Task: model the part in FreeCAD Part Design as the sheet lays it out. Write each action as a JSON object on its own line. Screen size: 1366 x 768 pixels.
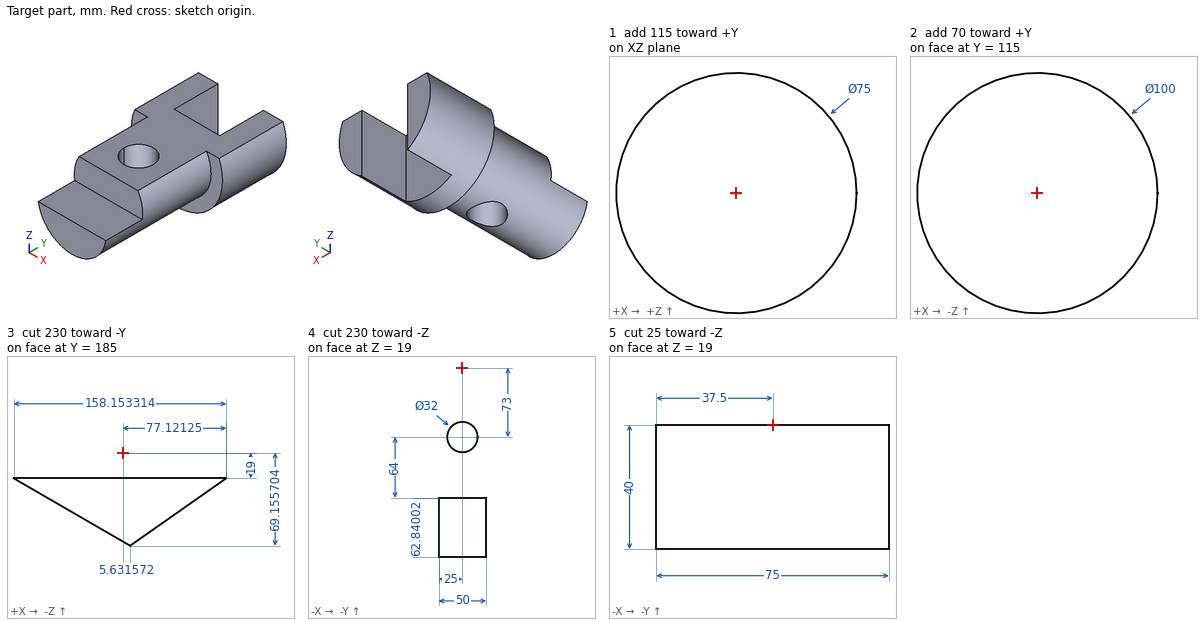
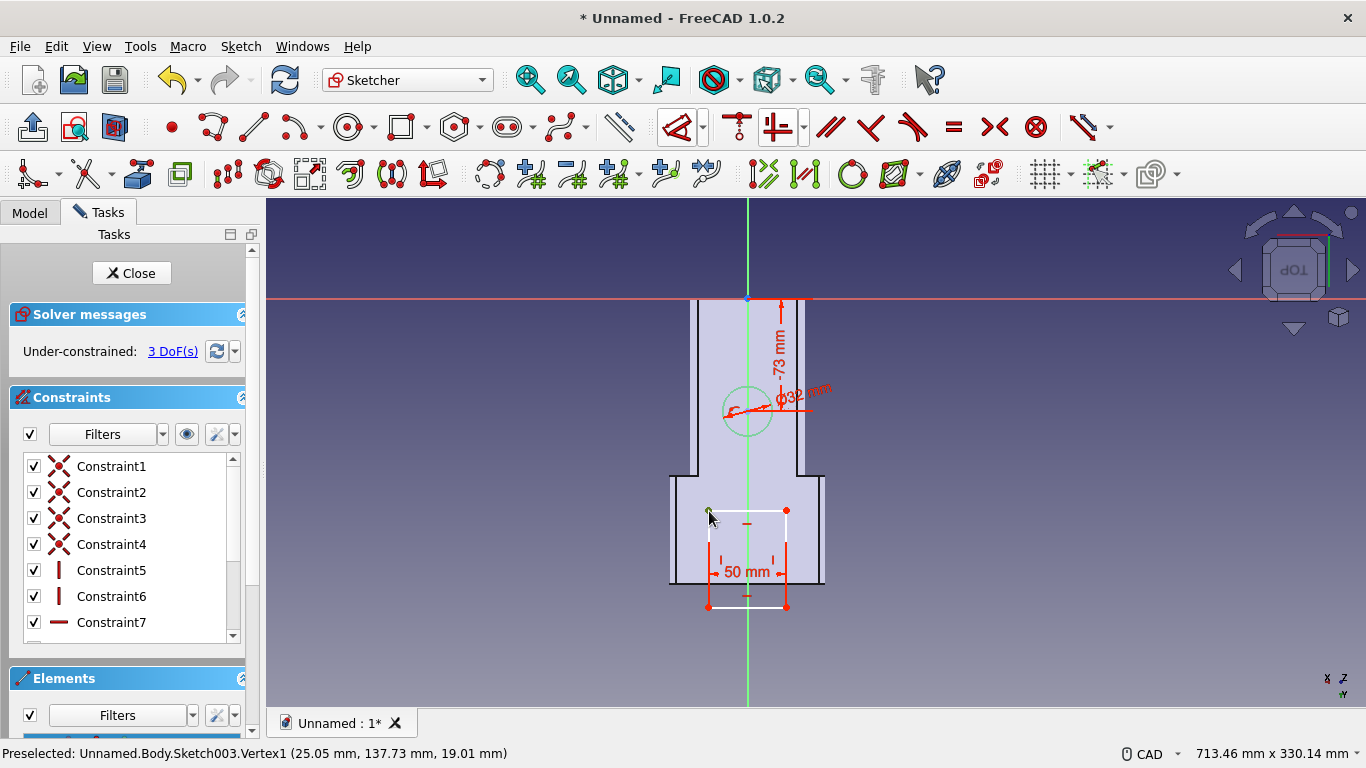
{"action": "key", "text": "l"}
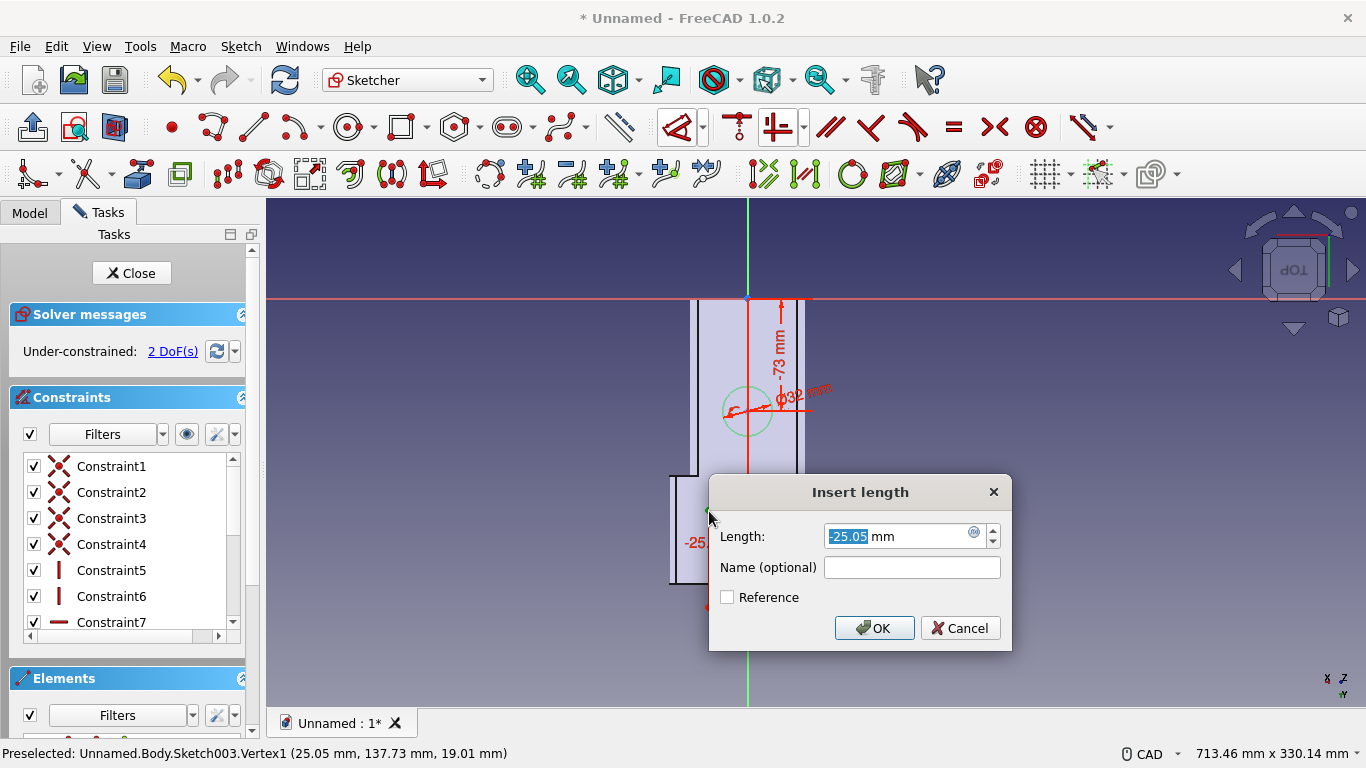
{"action": "type", "text": "-25"}
{"action": "key", "text": "Return"}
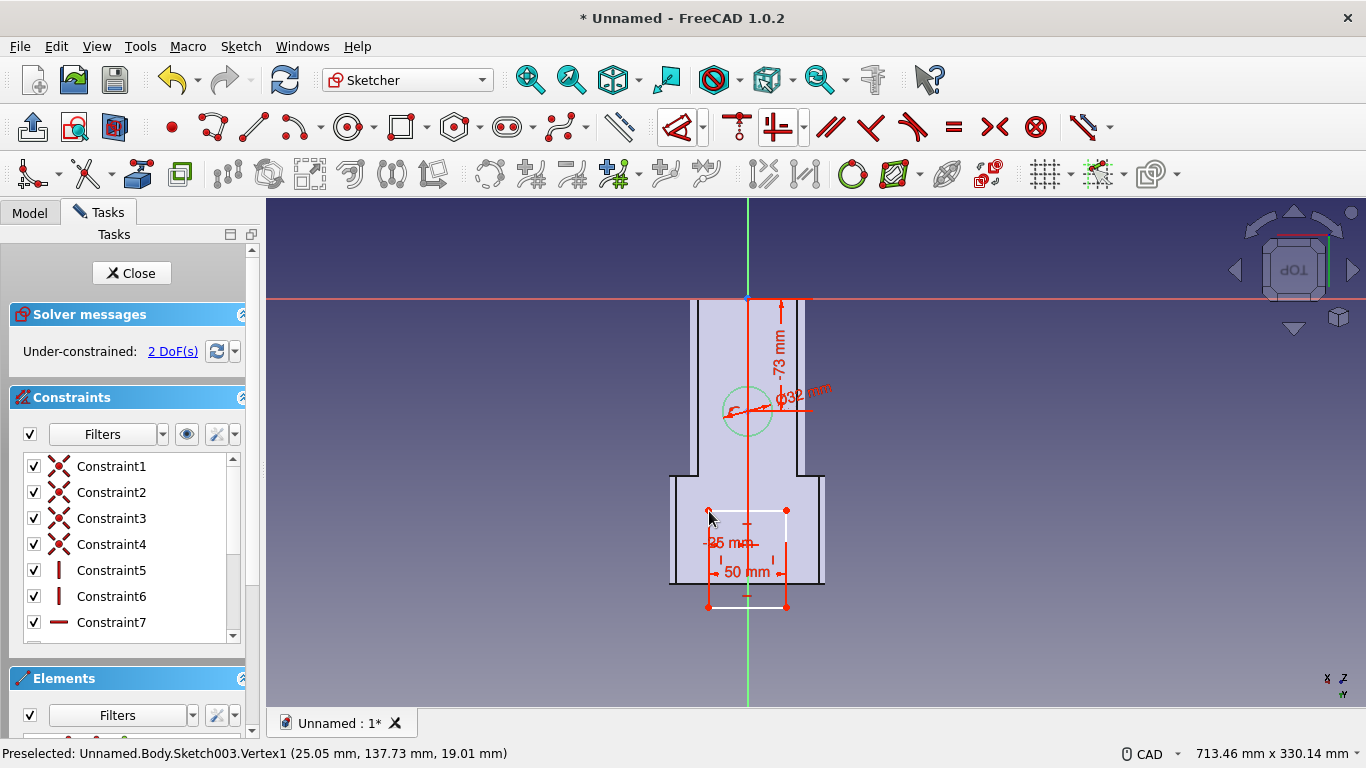
{"action": "left_click", "coordinate": [709, 511]}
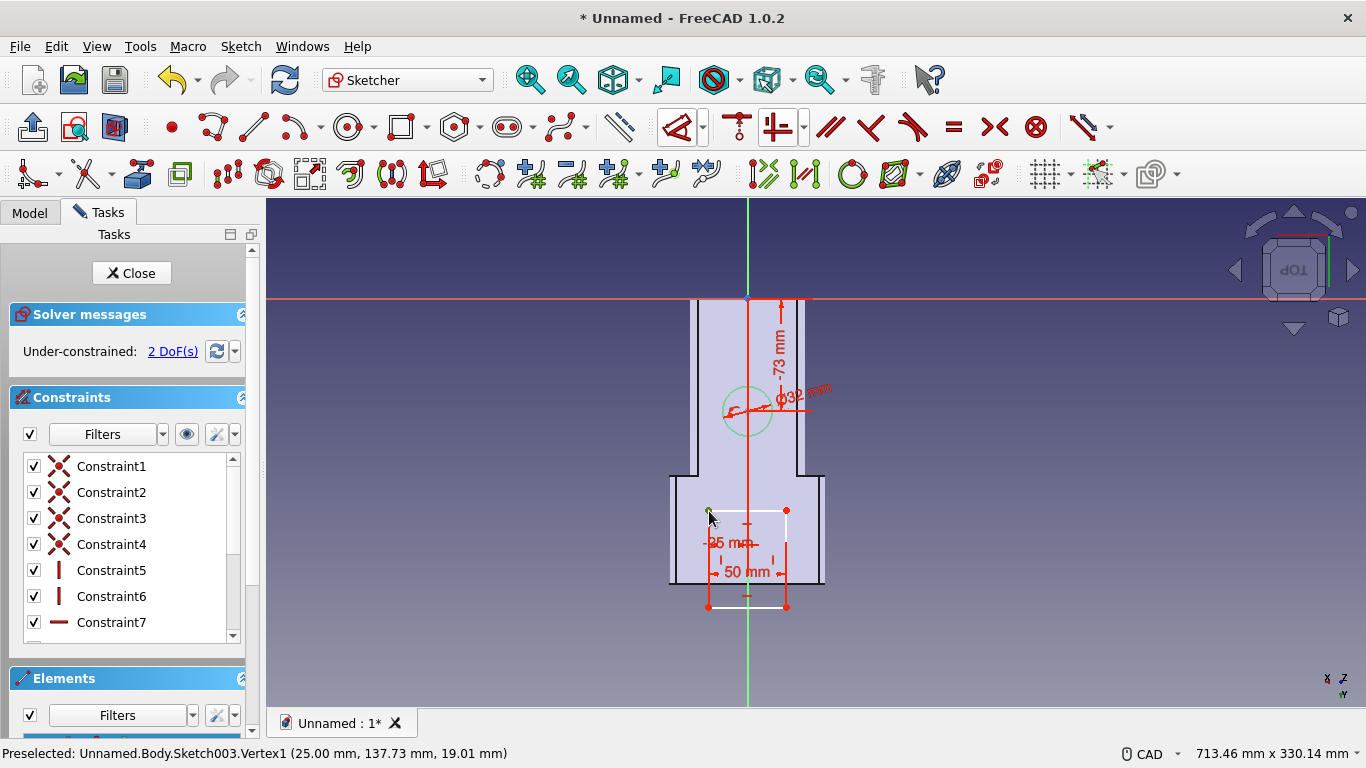
{"action": "left_click", "coordinate": [748, 411]}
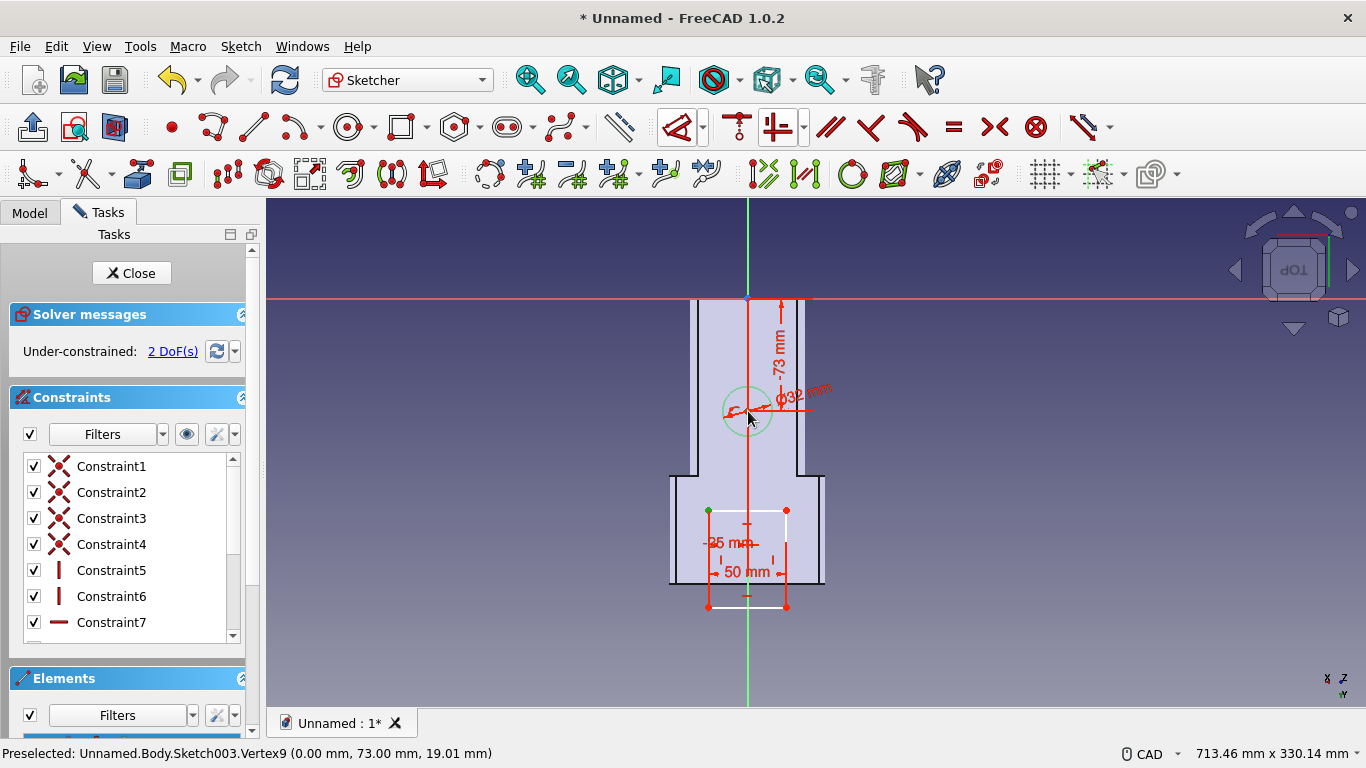
{"action": "left_click", "coordinate": [702, 128]}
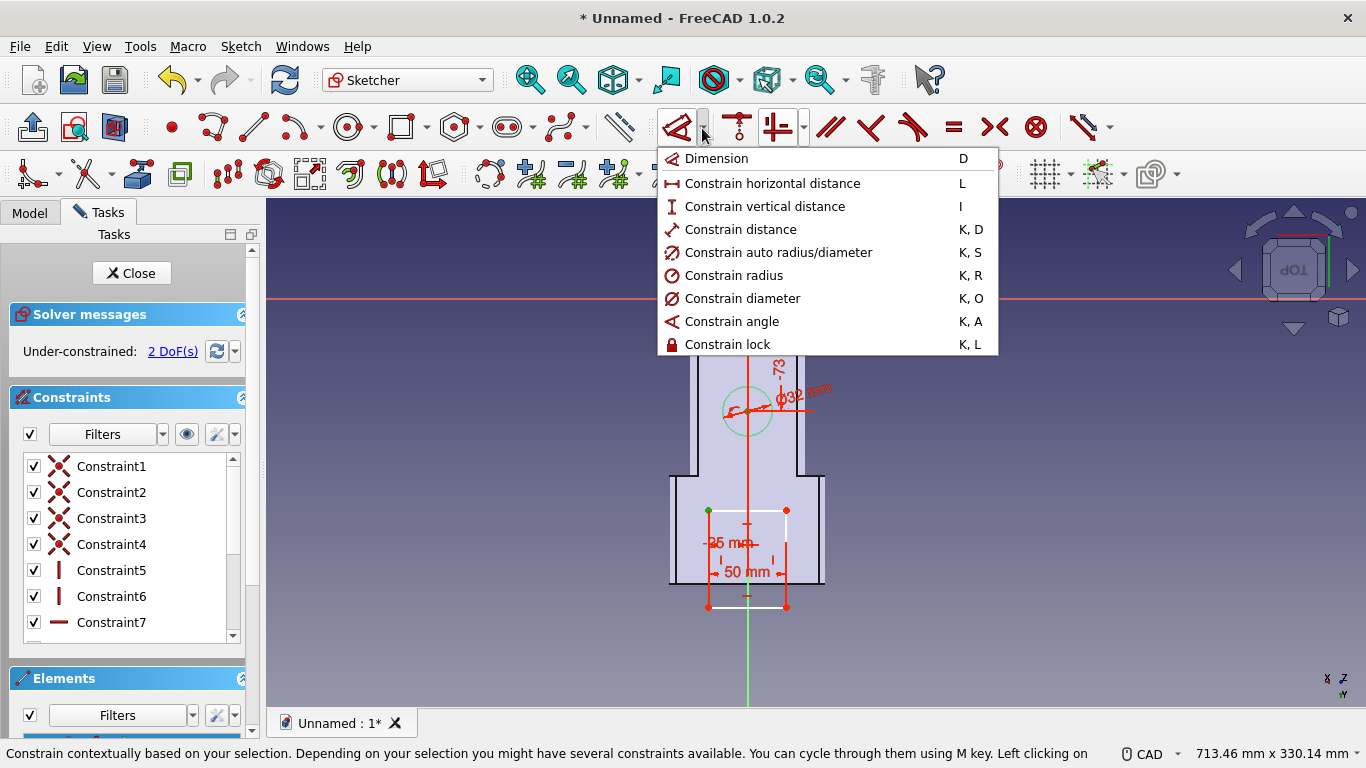
{"action": "left_click", "coordinate": [828, 206]}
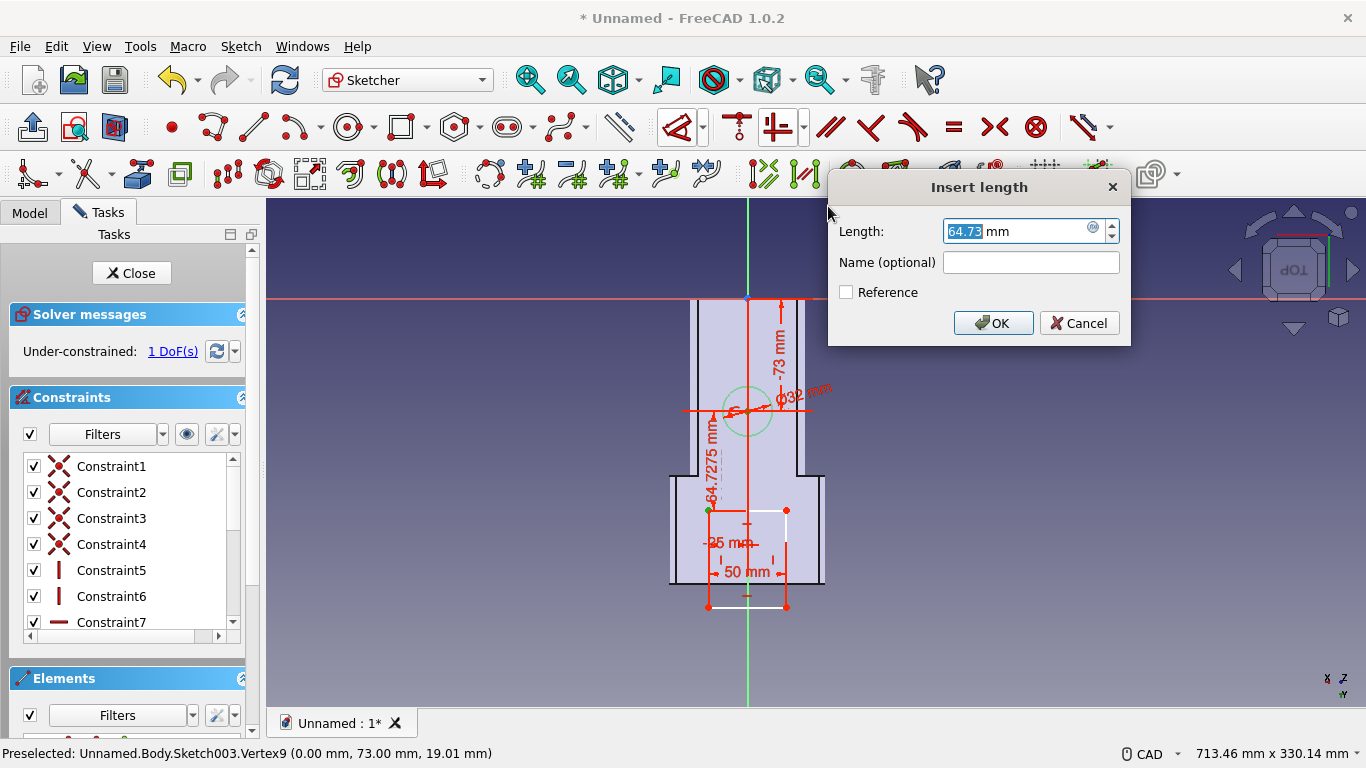
{"action": "type", "text": "64"}
{"action": "key", "text": "Return"}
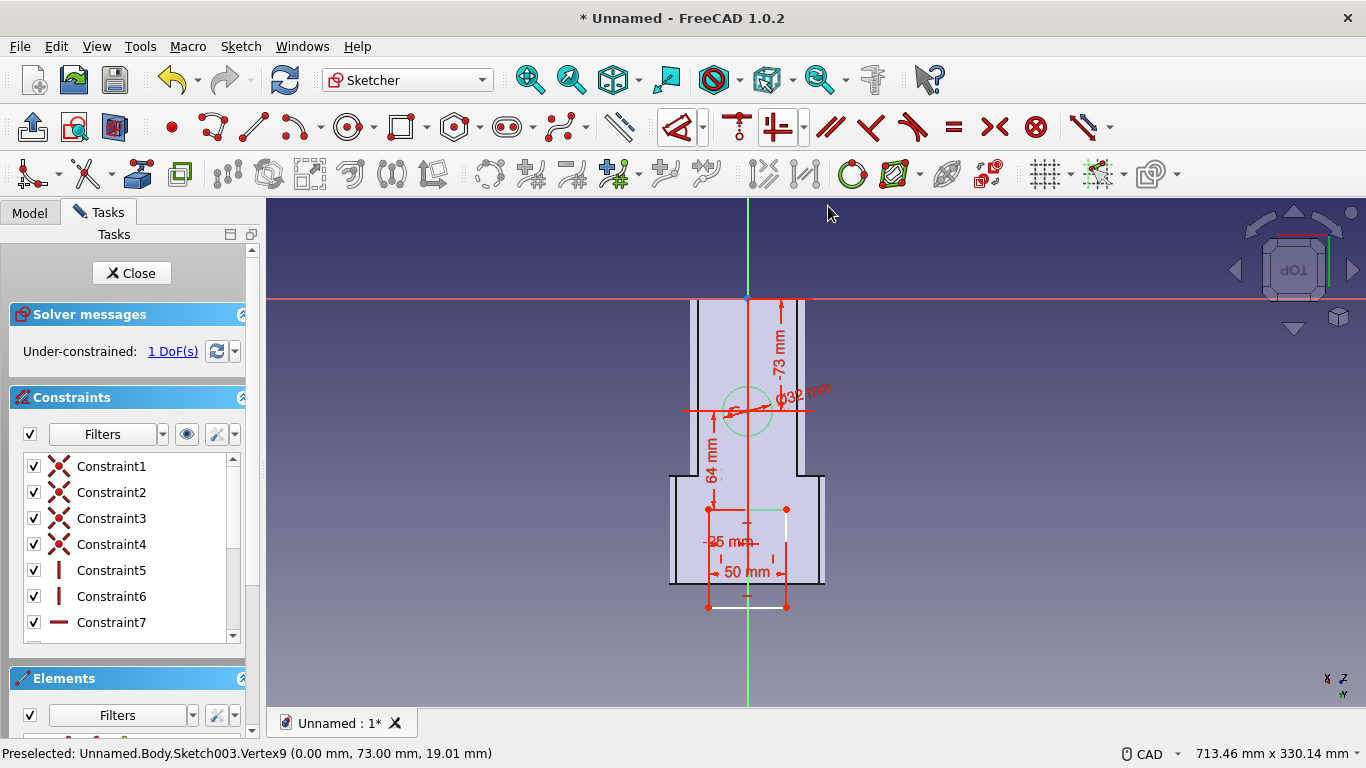
{"action": "left_click", "coordinate": [709, 579]}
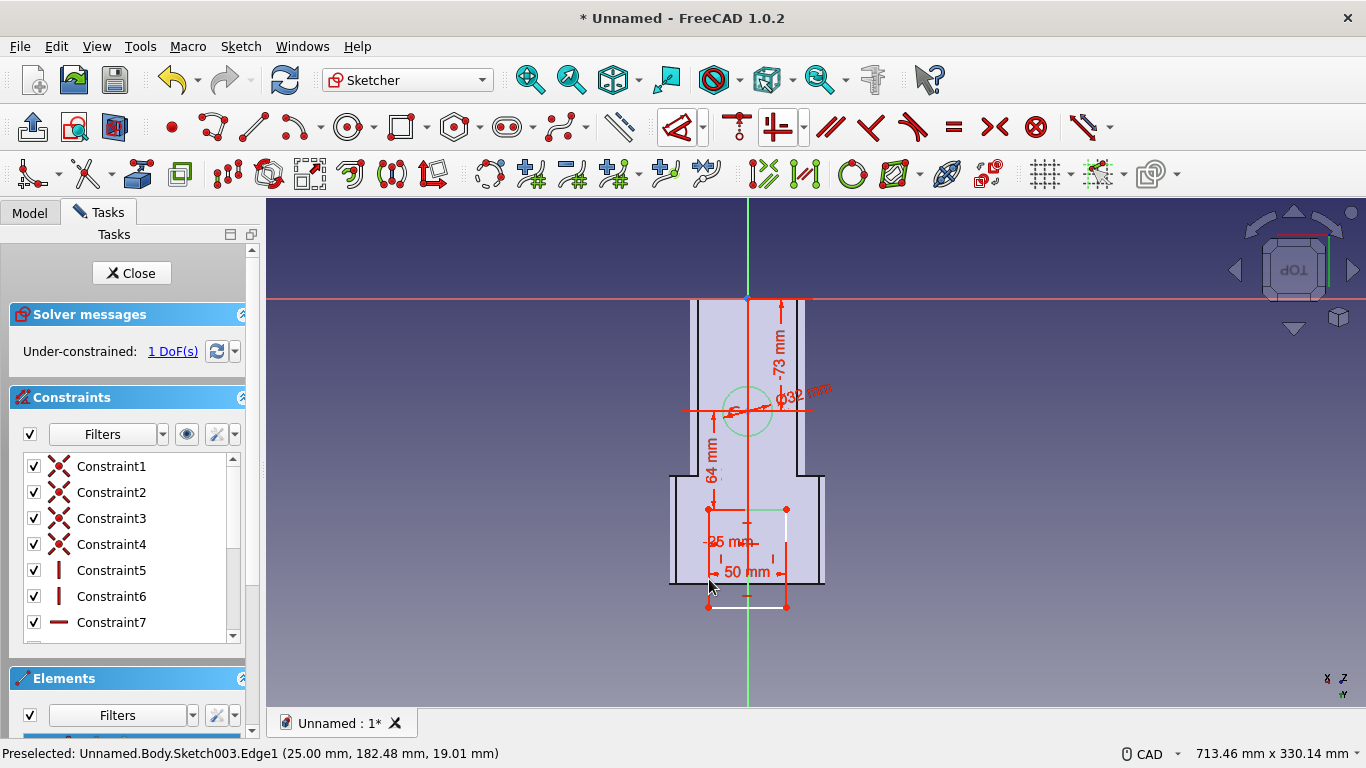
{"action": "left_click", "coordinate": [702, 128]}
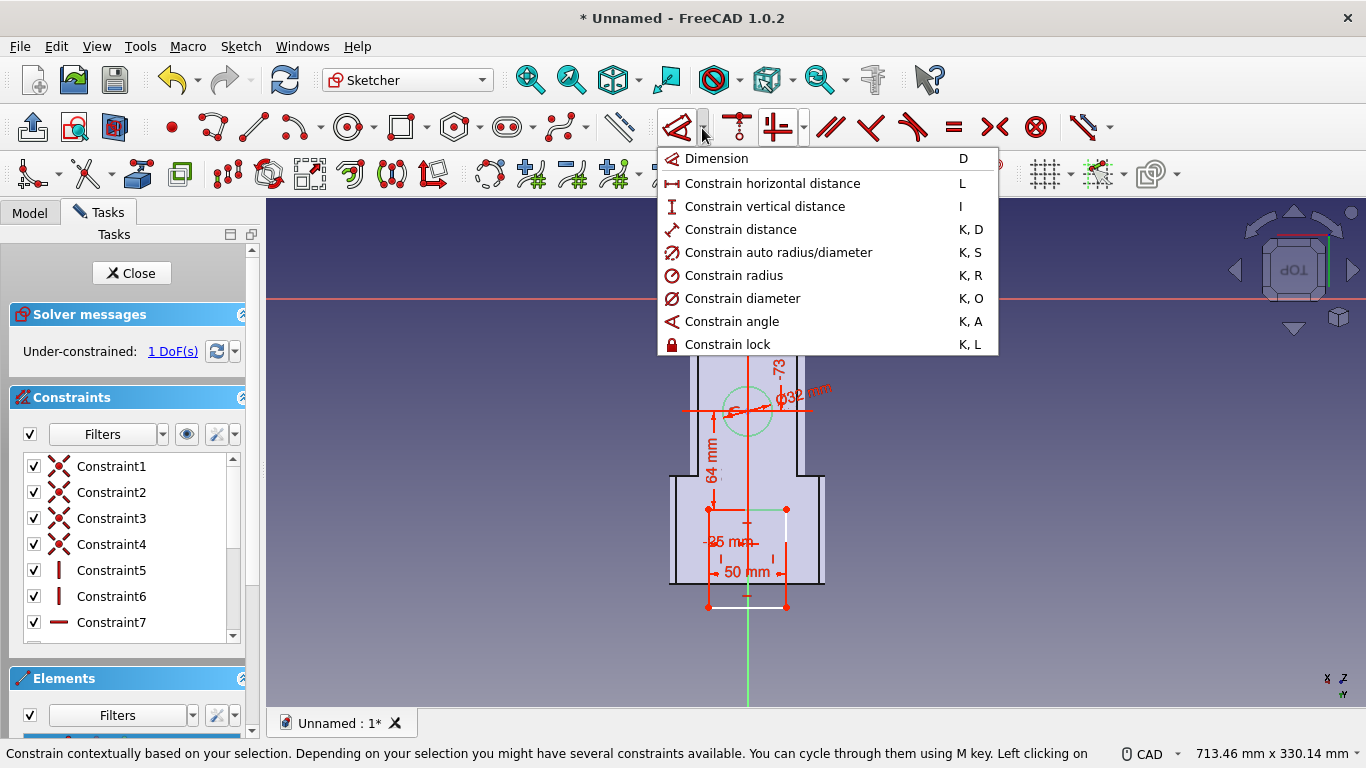
{"action": "left_click", "coordinate": [828, 206]}